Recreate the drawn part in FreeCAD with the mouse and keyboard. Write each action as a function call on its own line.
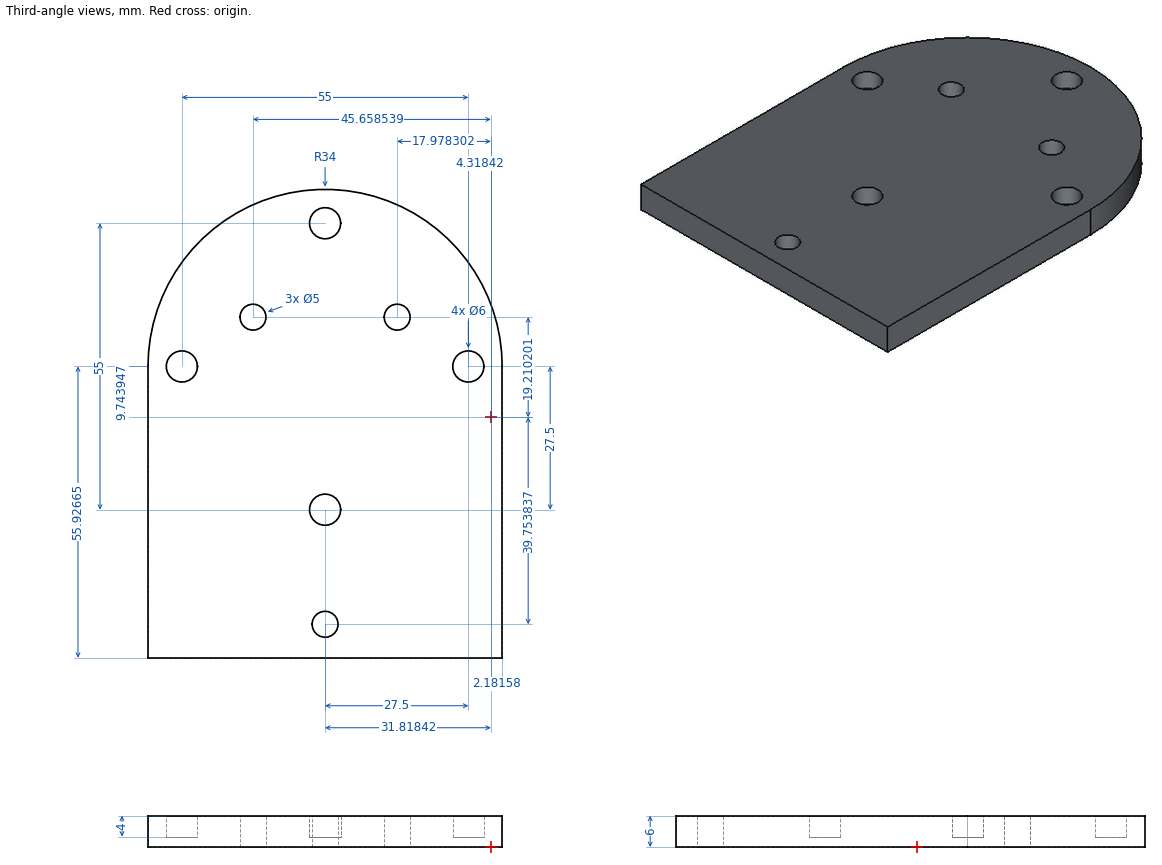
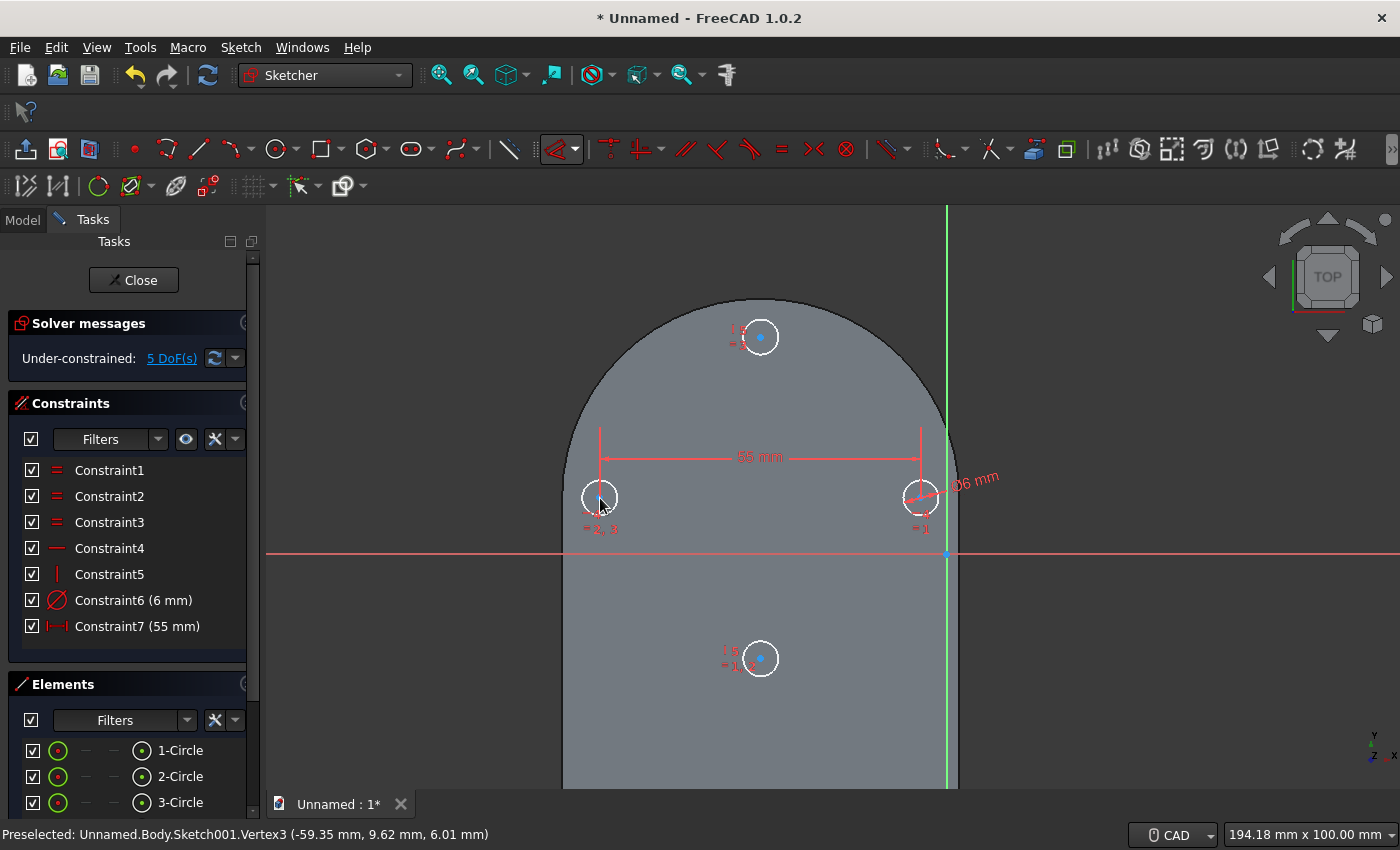
click(761, 659)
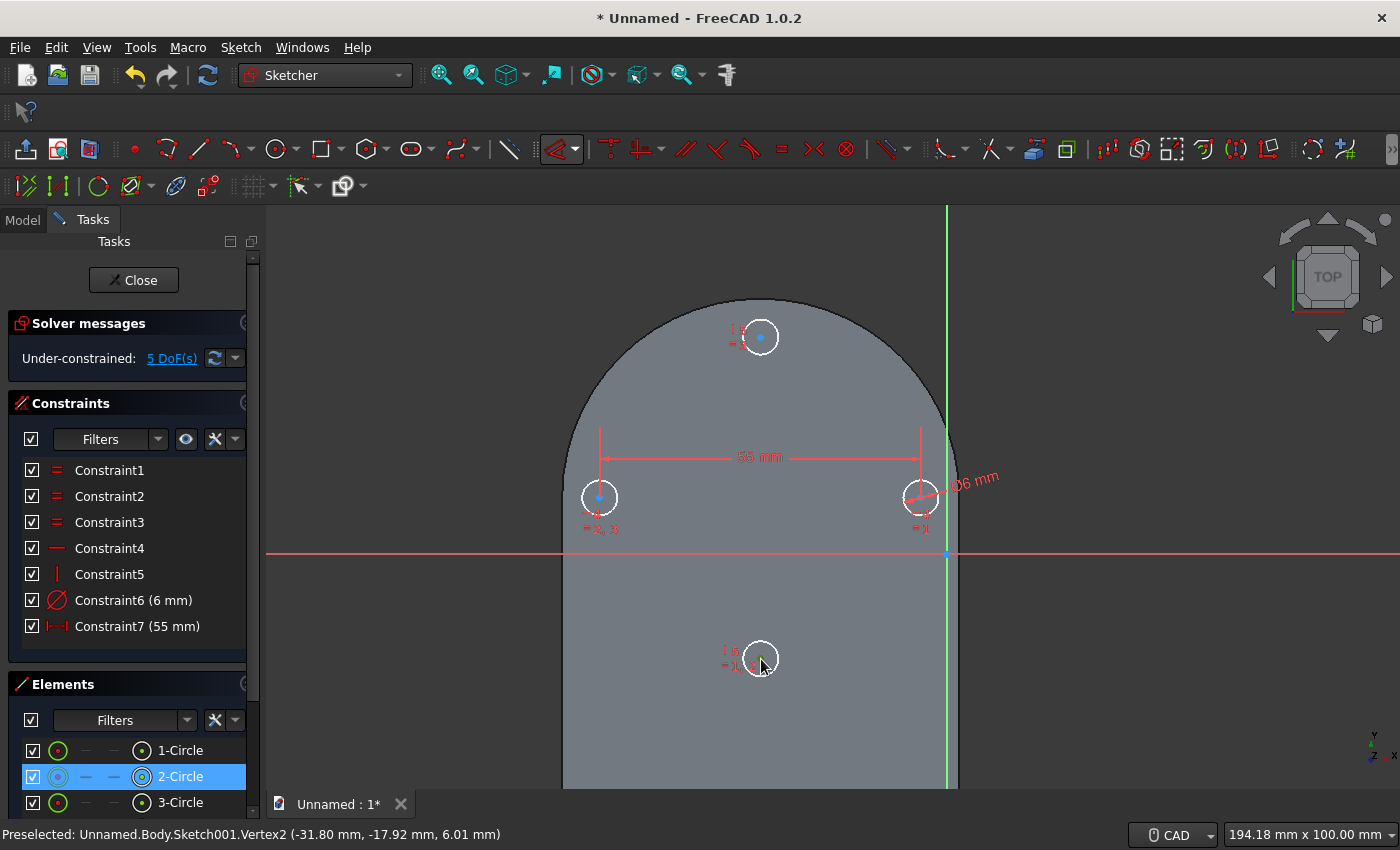
click(761, 337)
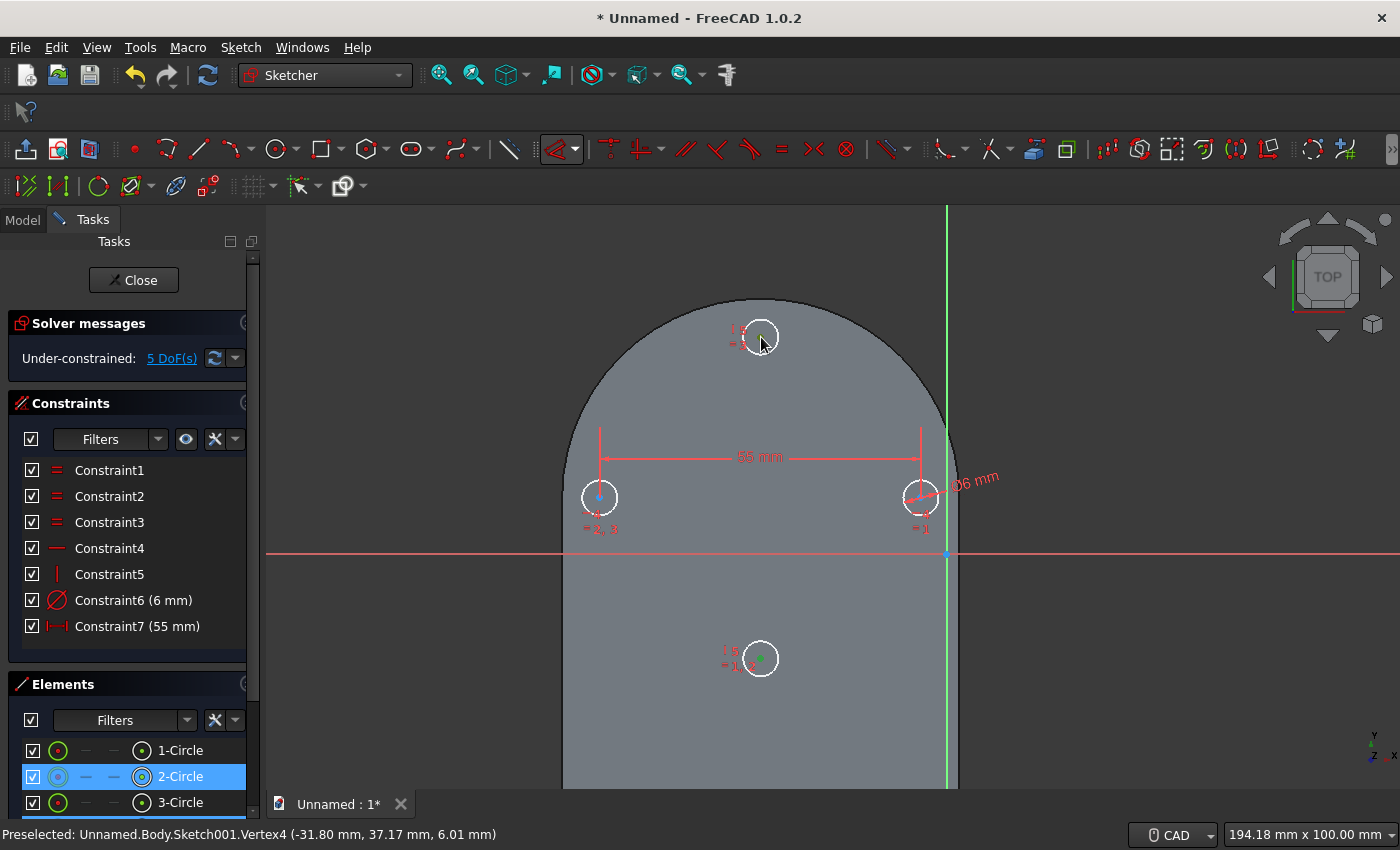
key(i)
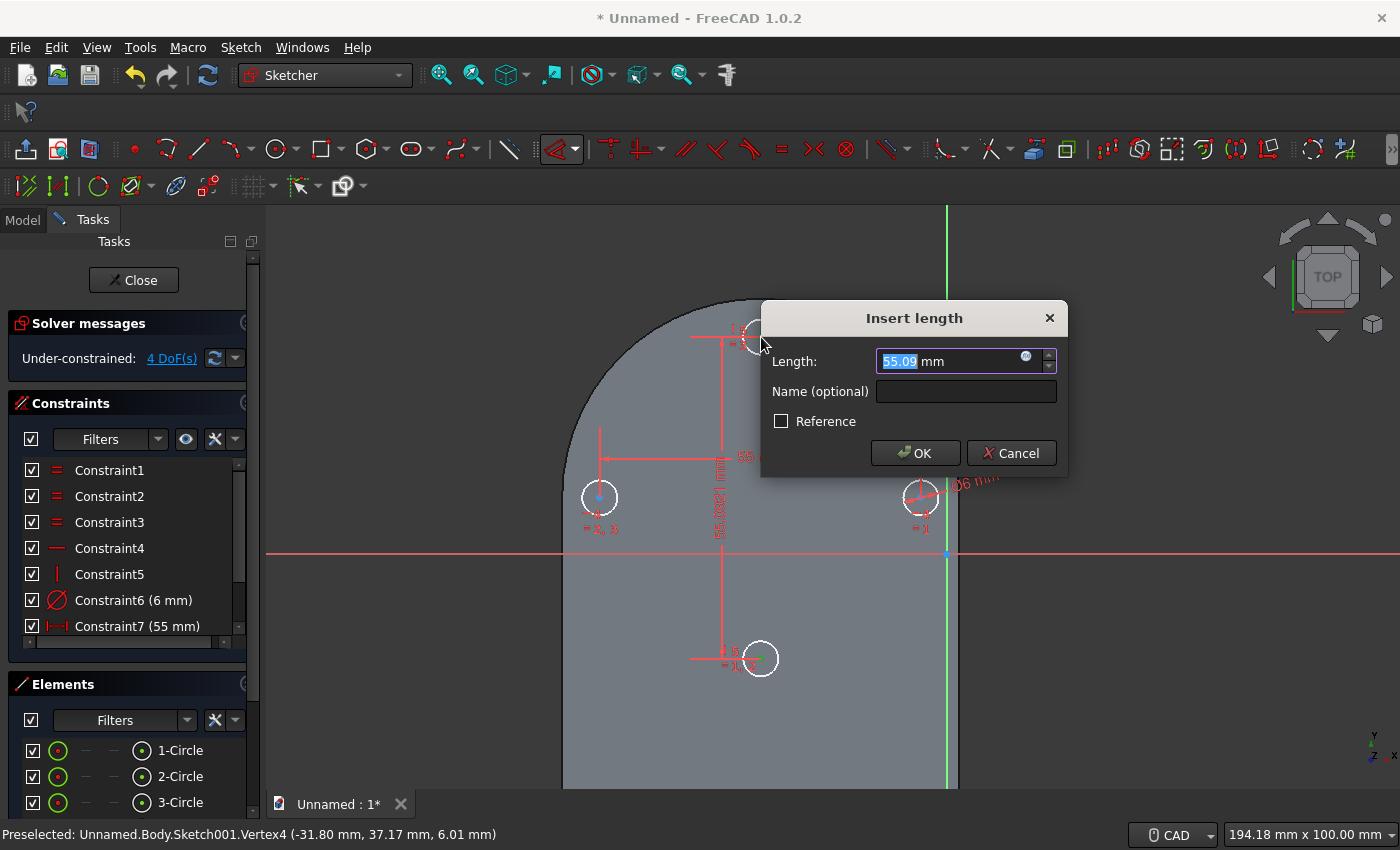
text(55)
key(Return)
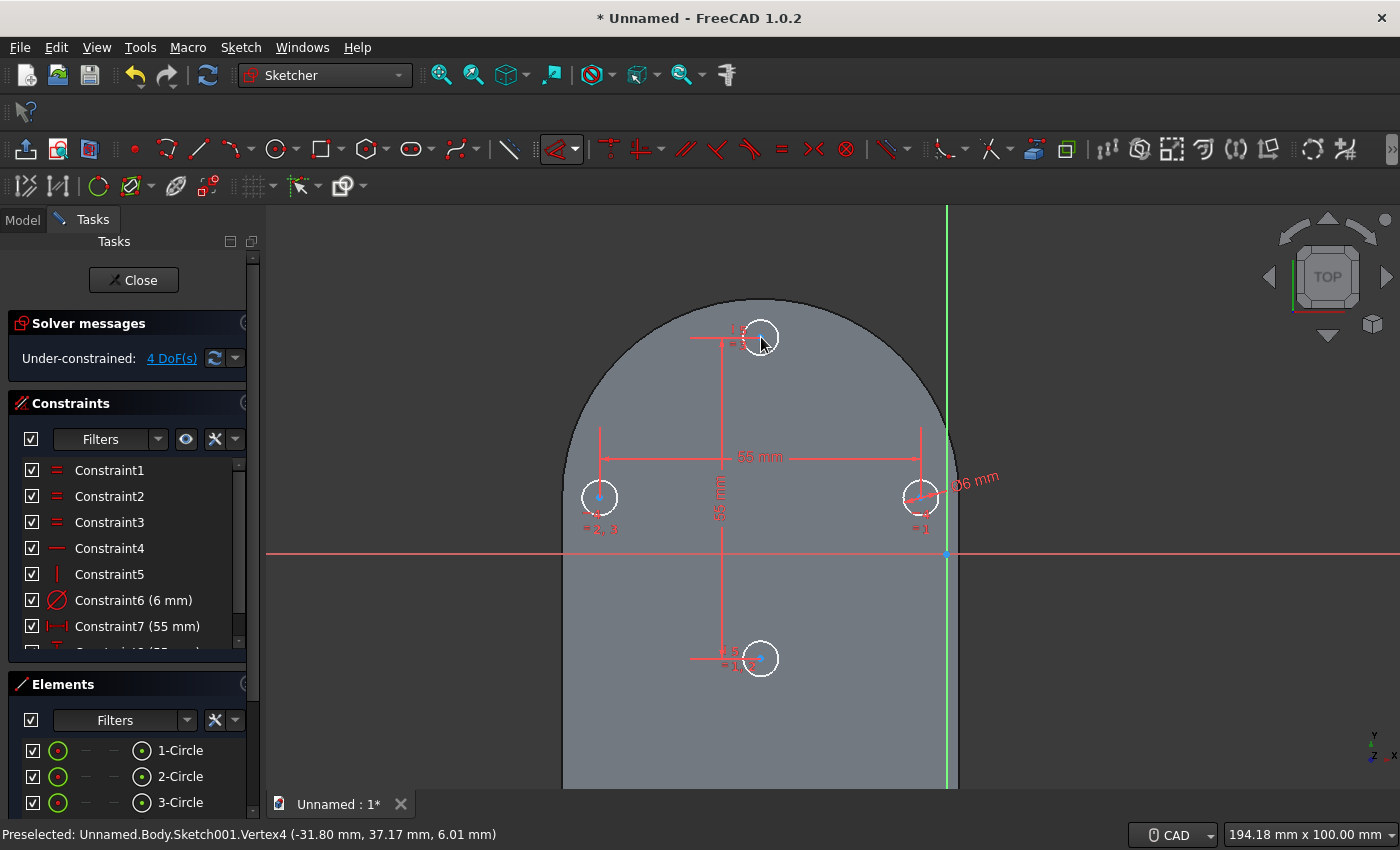
click(921, 498)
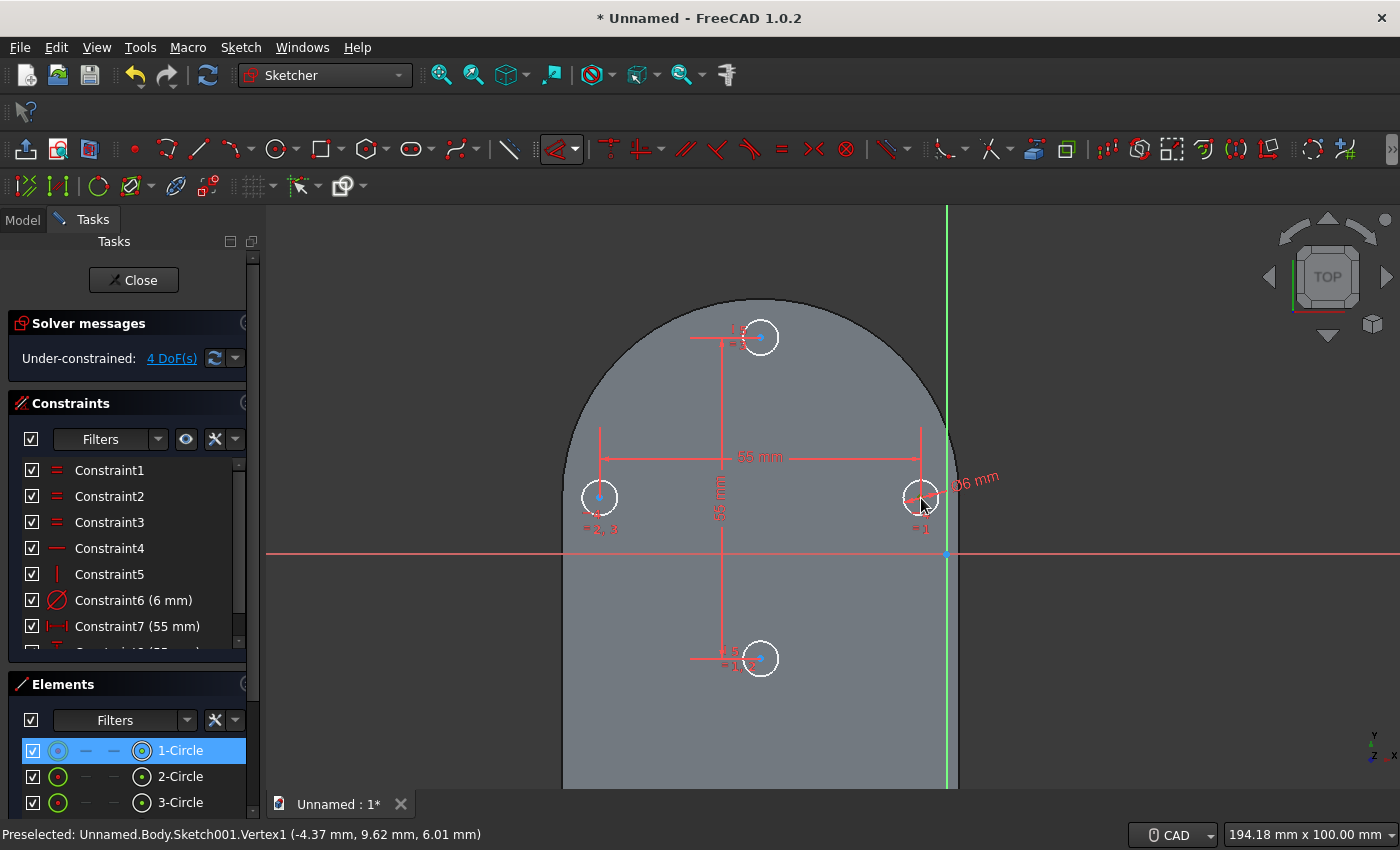
click(761, 659)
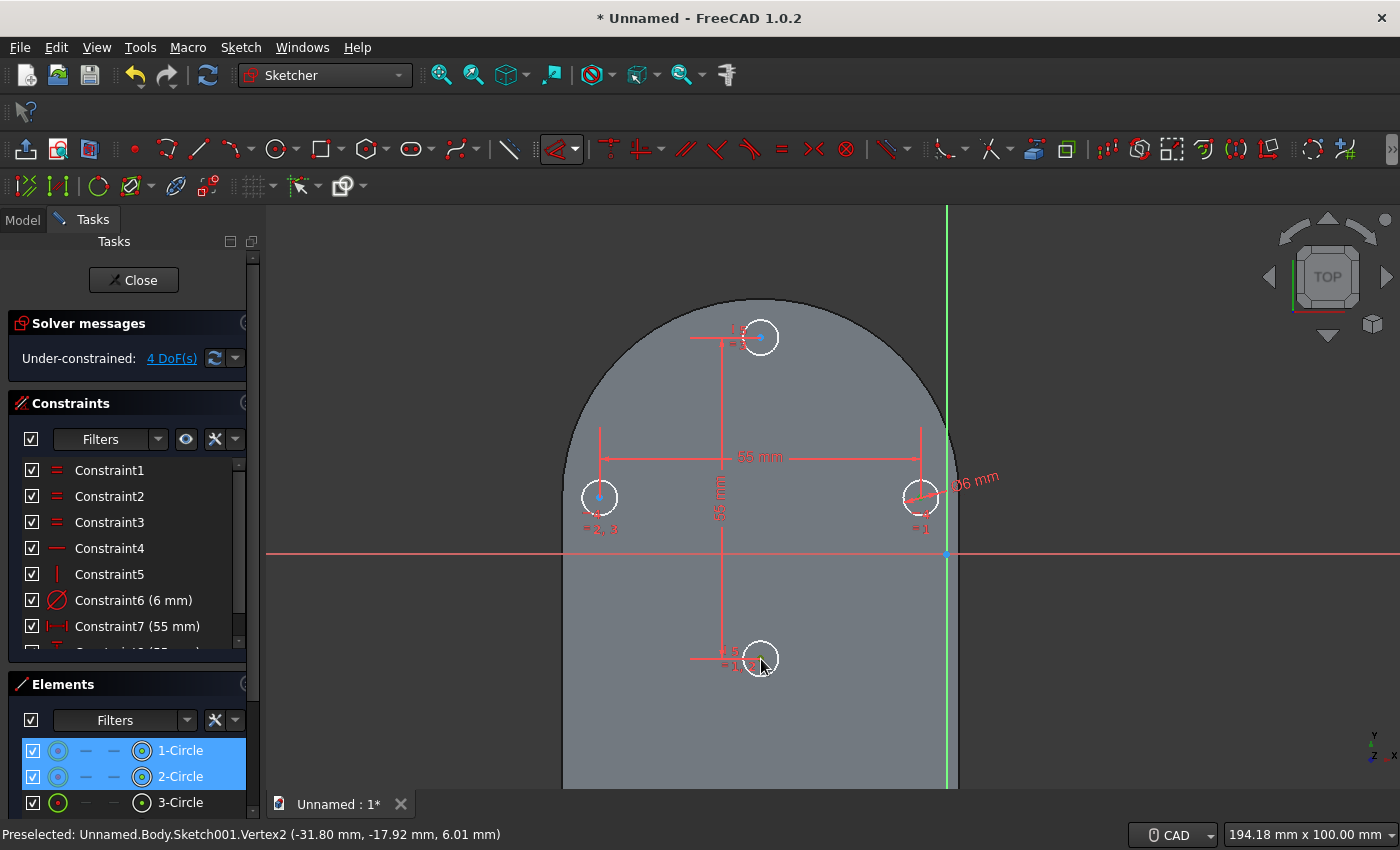
key(l)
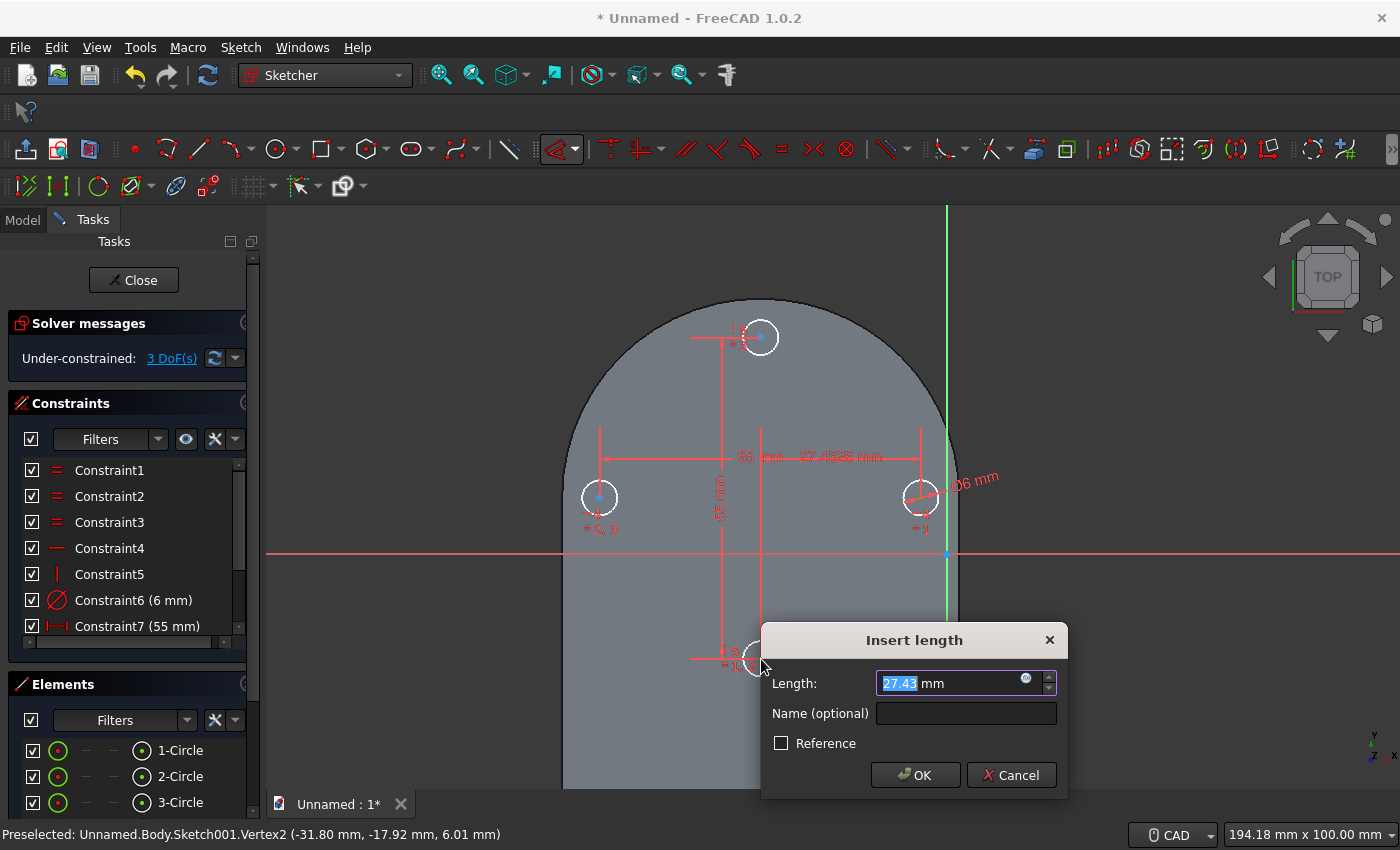
text(27.5)
key(Return)